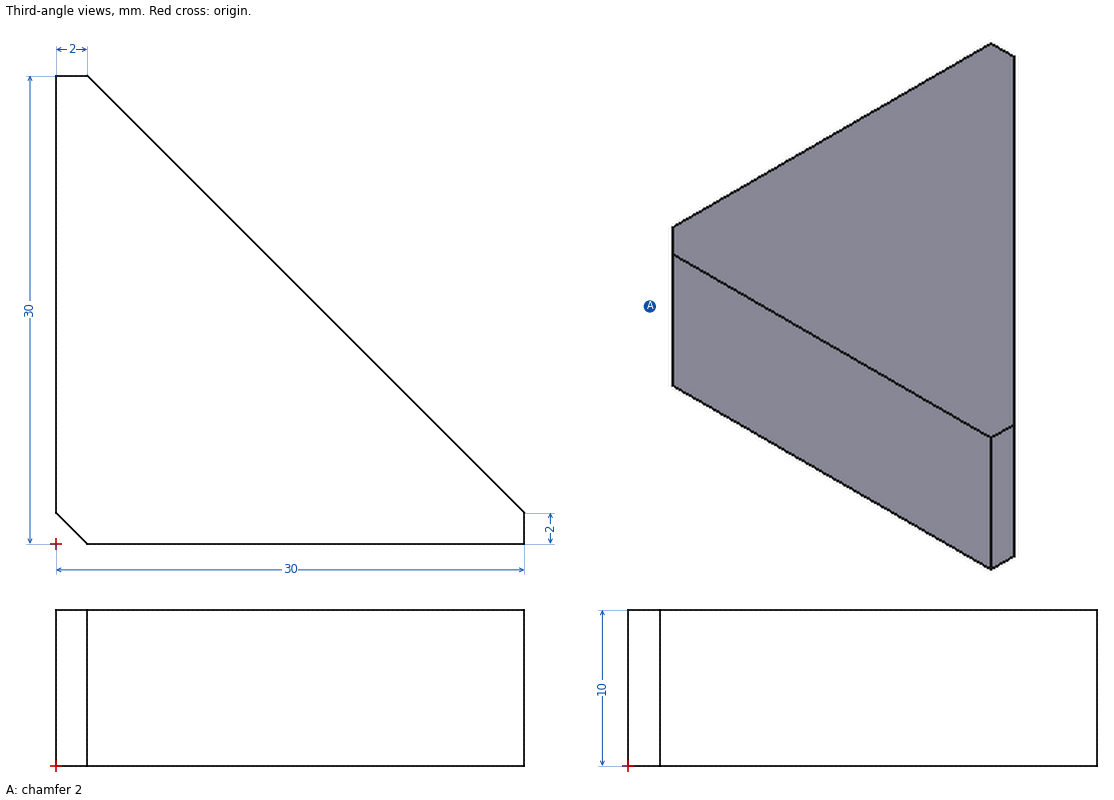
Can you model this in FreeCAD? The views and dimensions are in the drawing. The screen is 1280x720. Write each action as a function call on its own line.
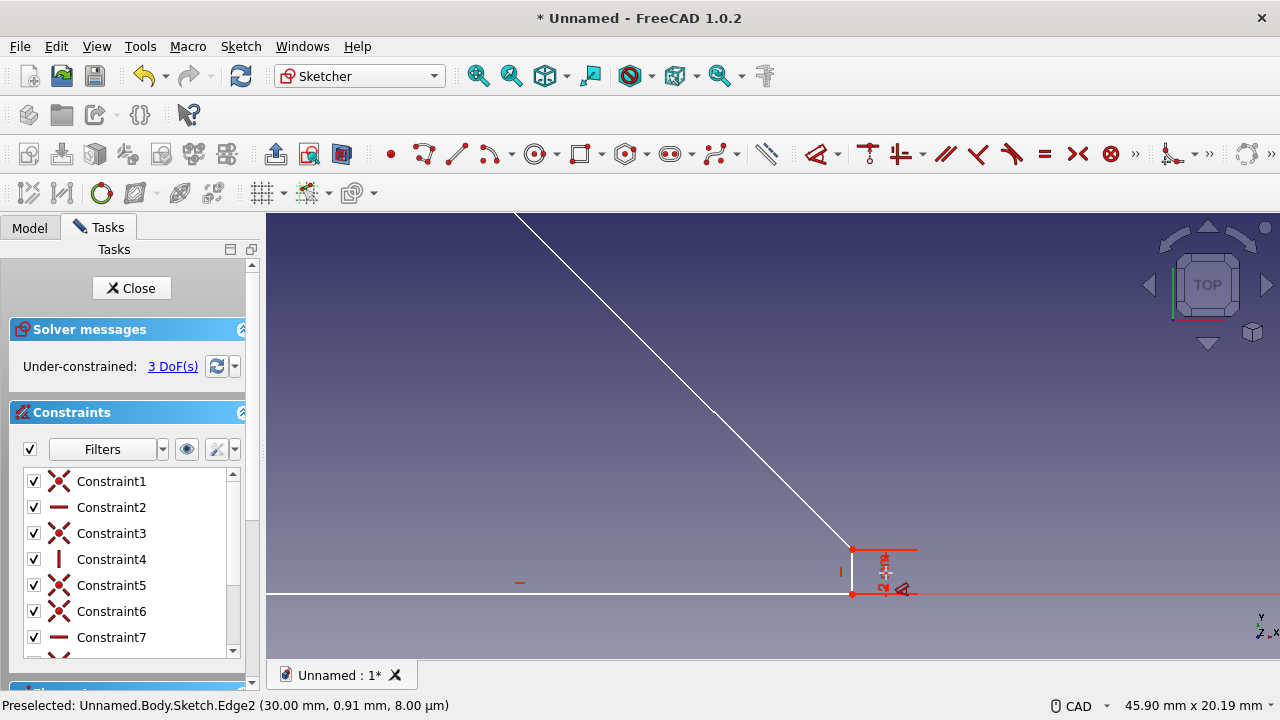
scroll(854, 577, down, 4)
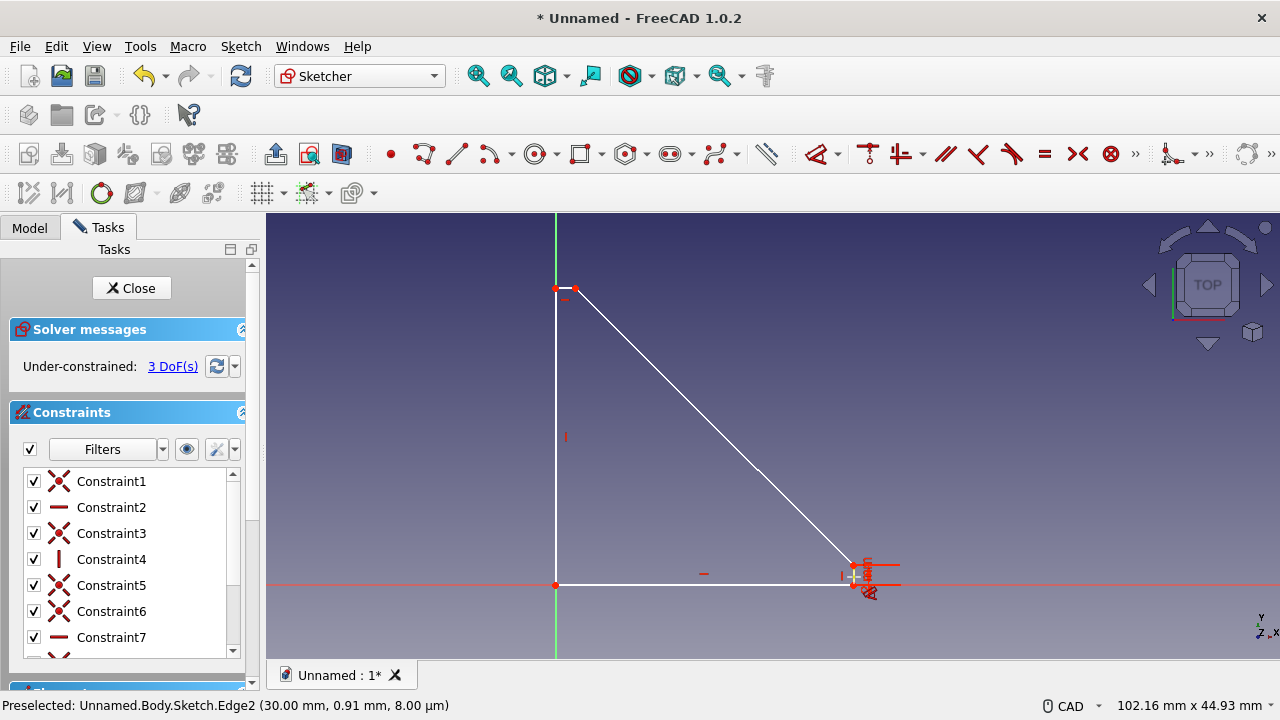
scroll(570, 288, up, 5)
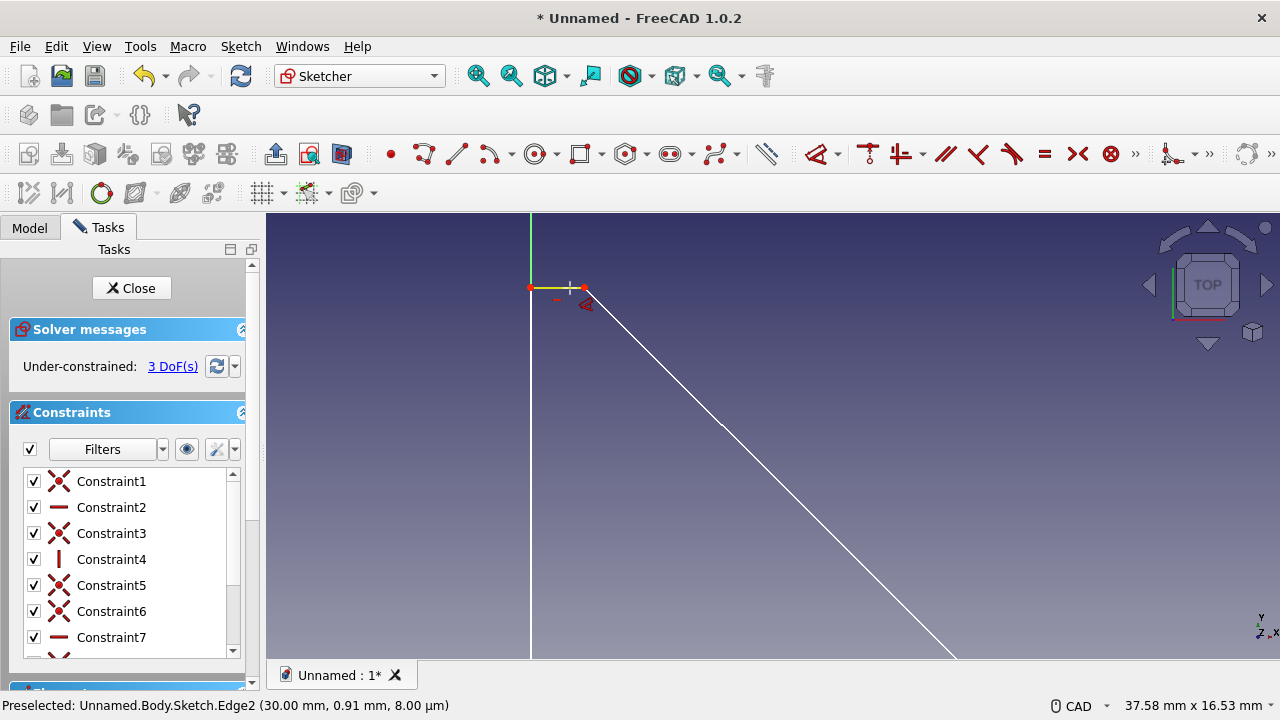
click(568, 288)
click(558, 254)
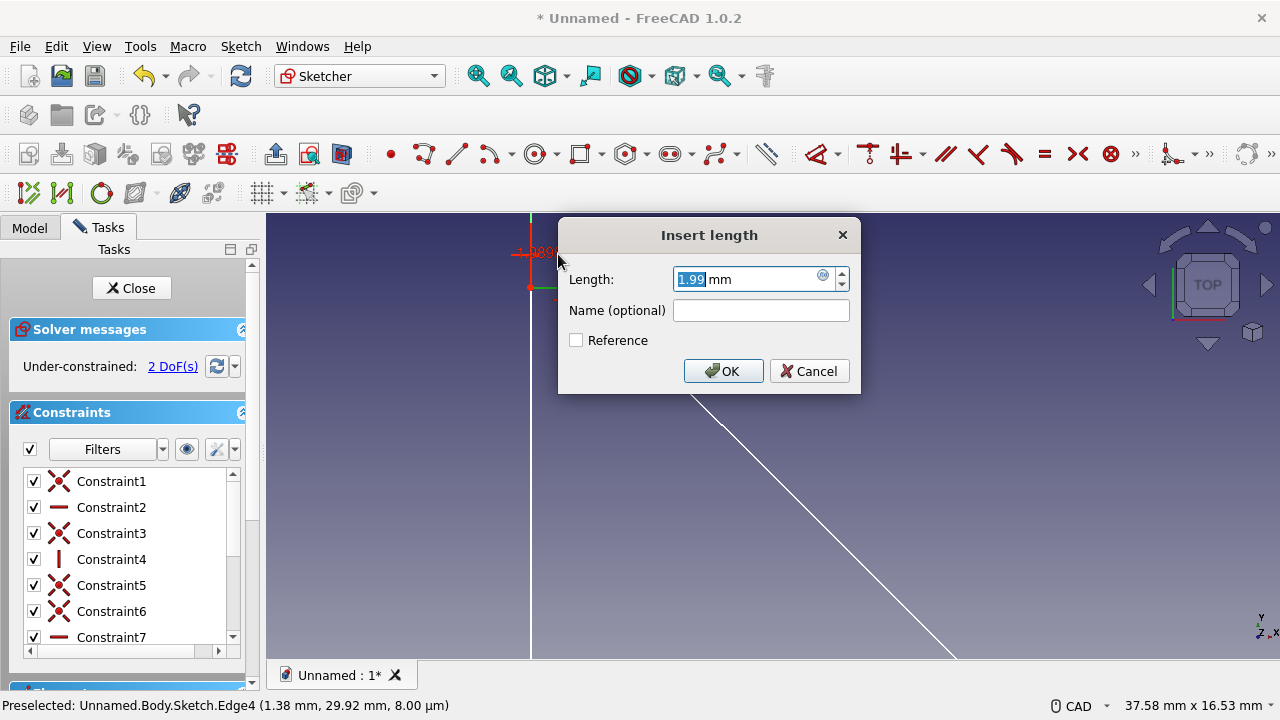
text(2)
key(Return)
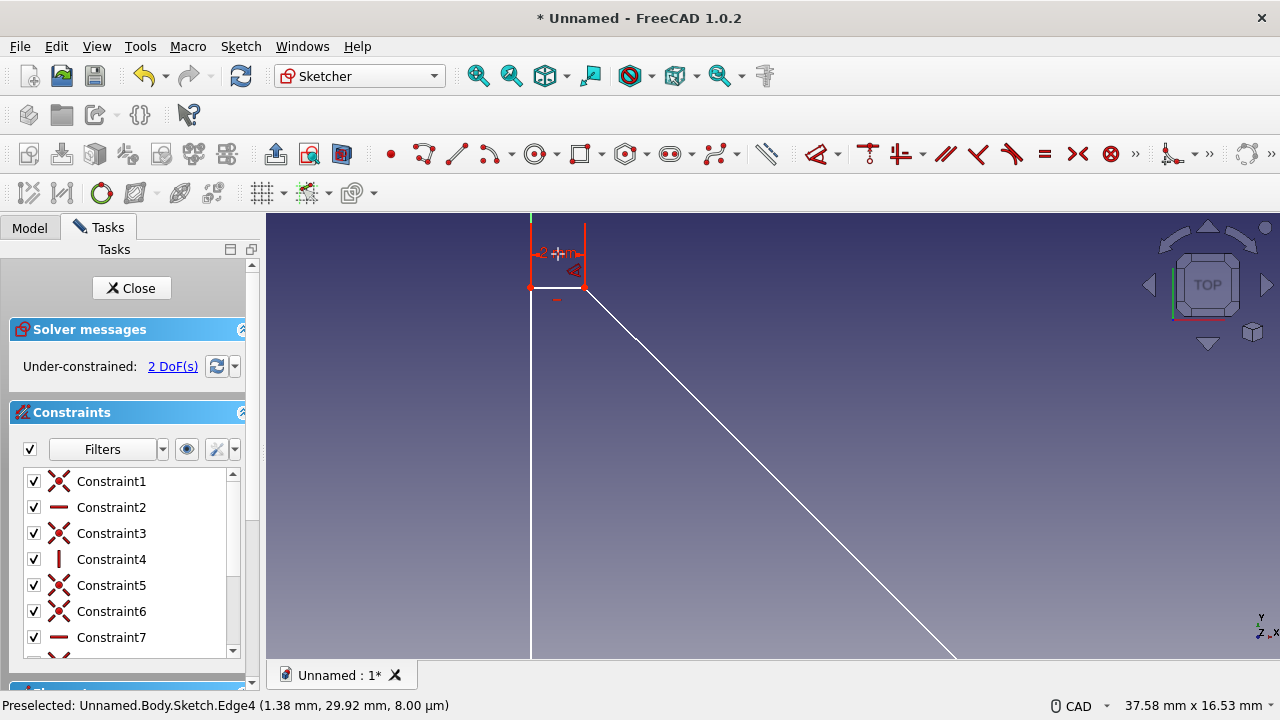
scroll(570, 288, down, 5)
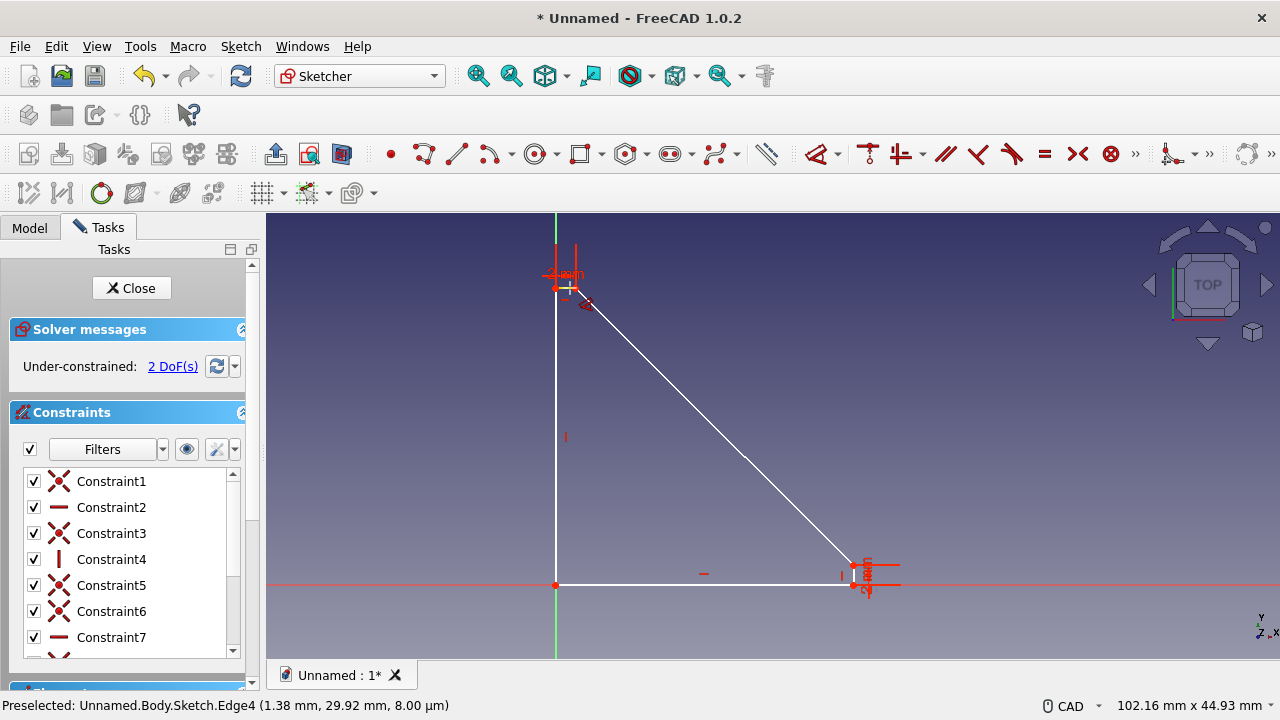
click(645, 585)
click(705, 619)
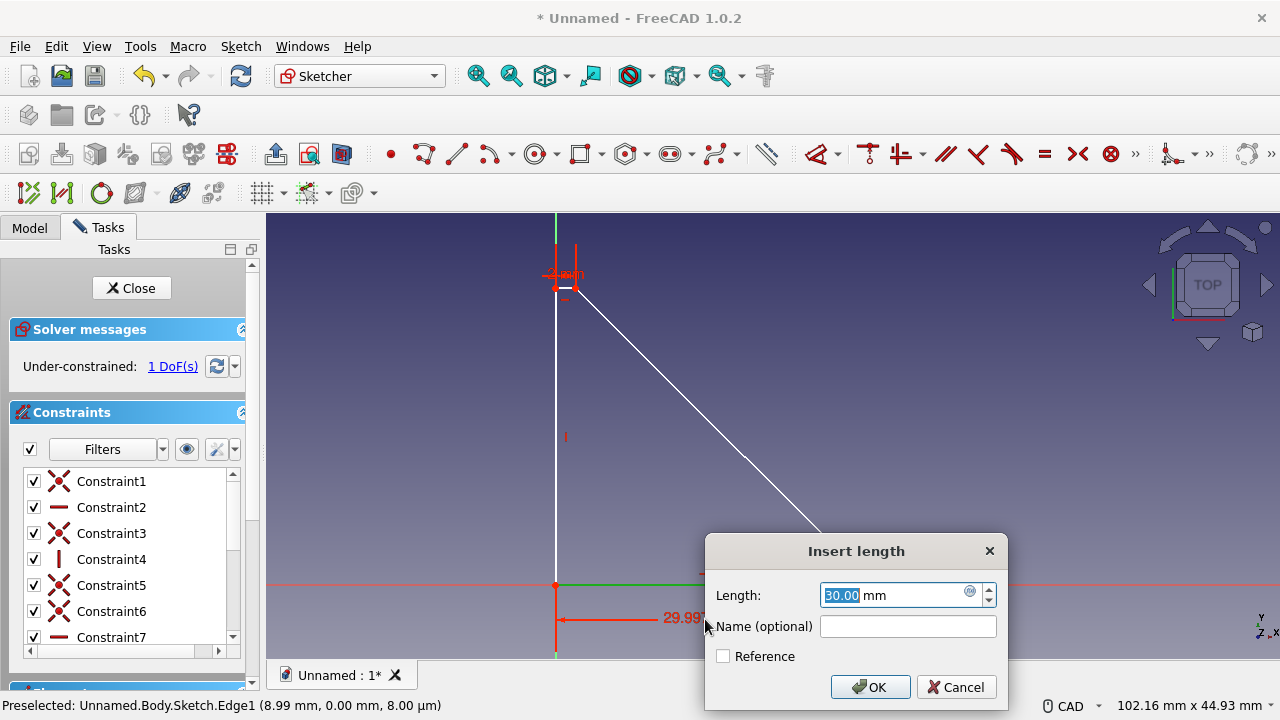
text(30)
key(Return)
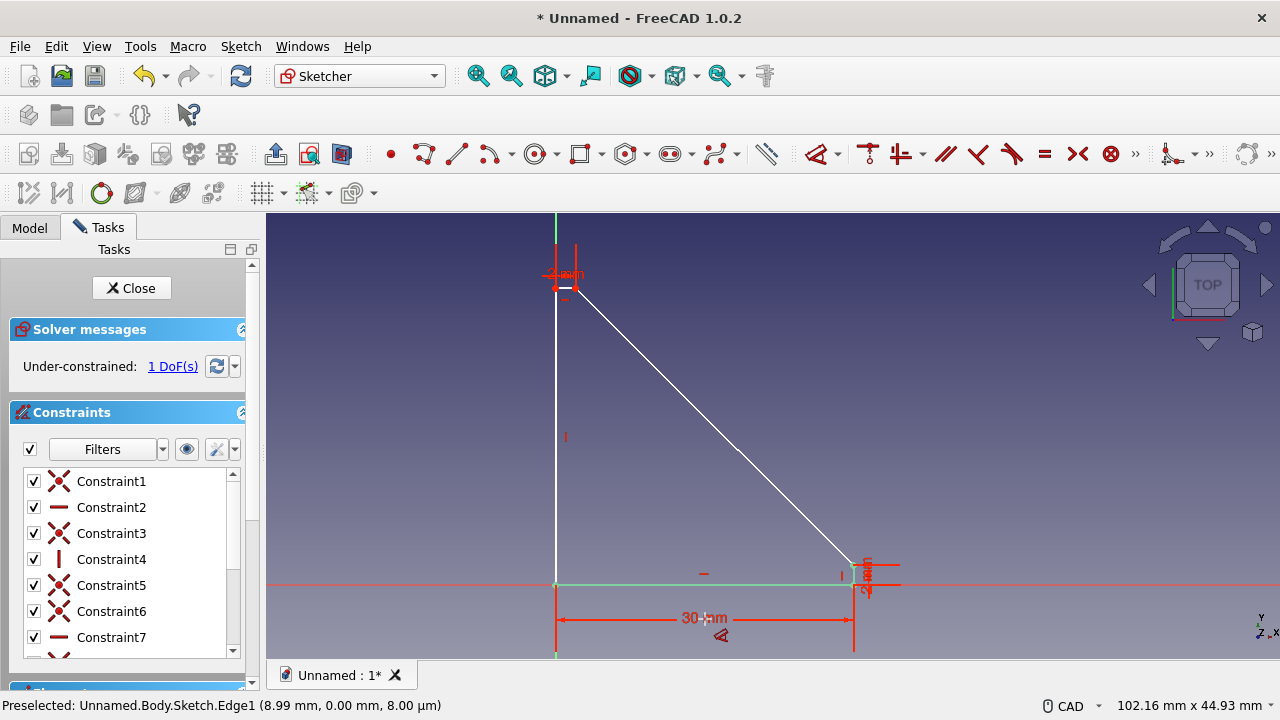
click(556, 377)
click(522, 437)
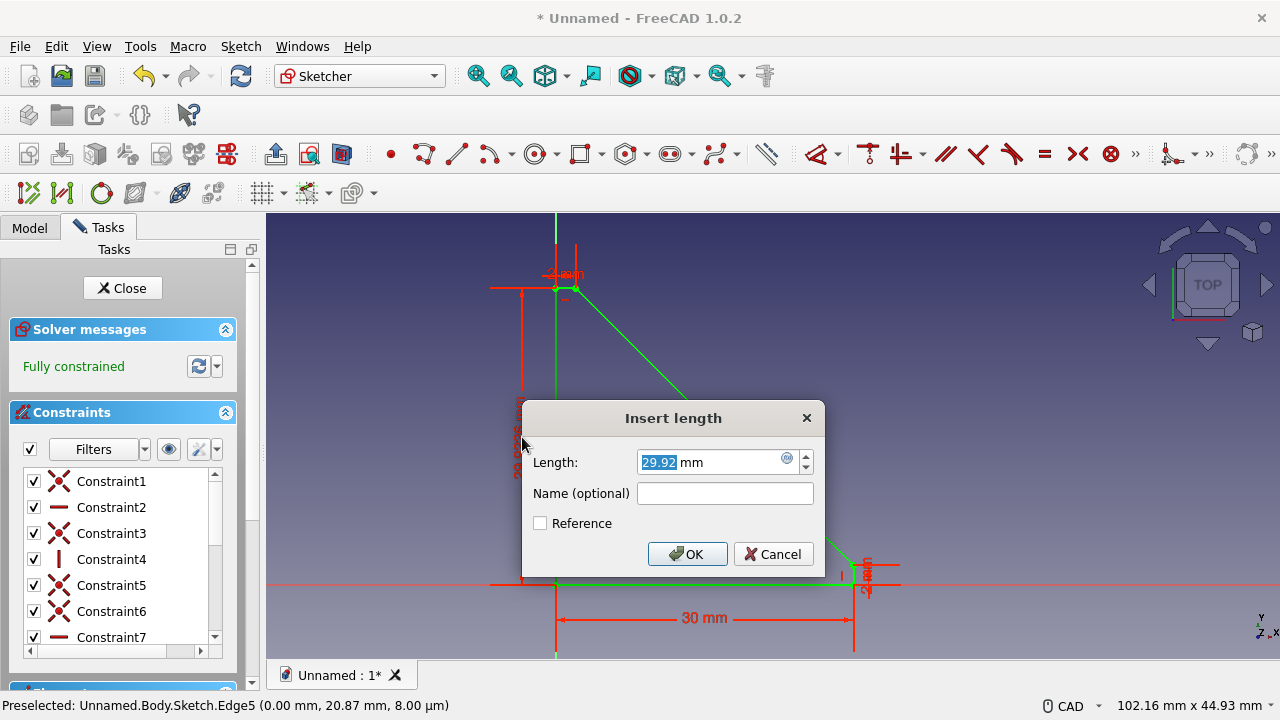
text(30)
key(Return)
key(Escape)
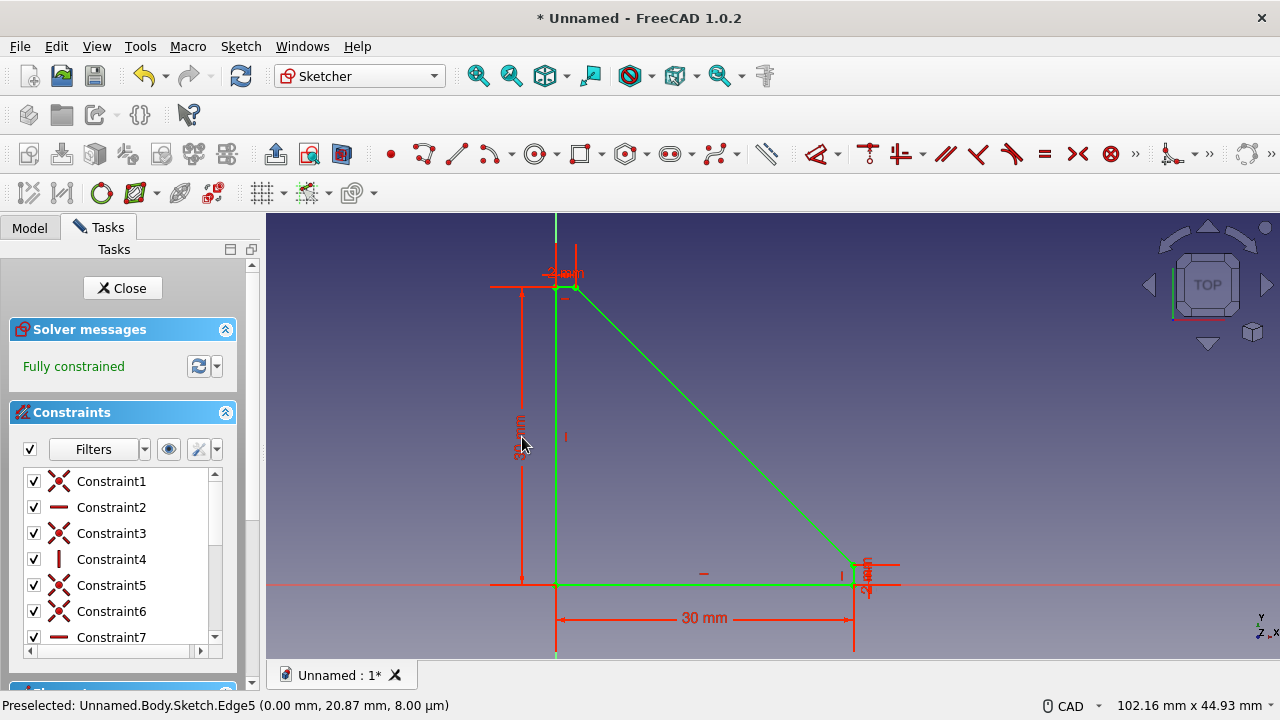
click(123, 288)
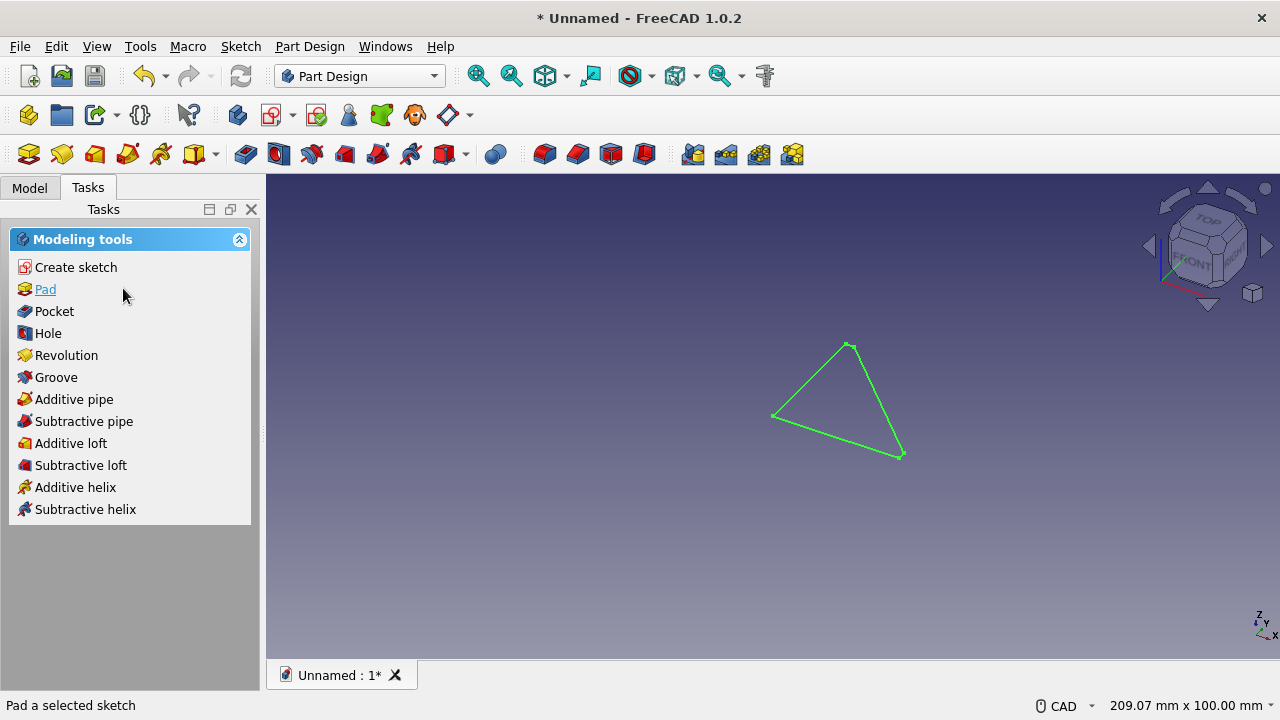
click(29, 154)